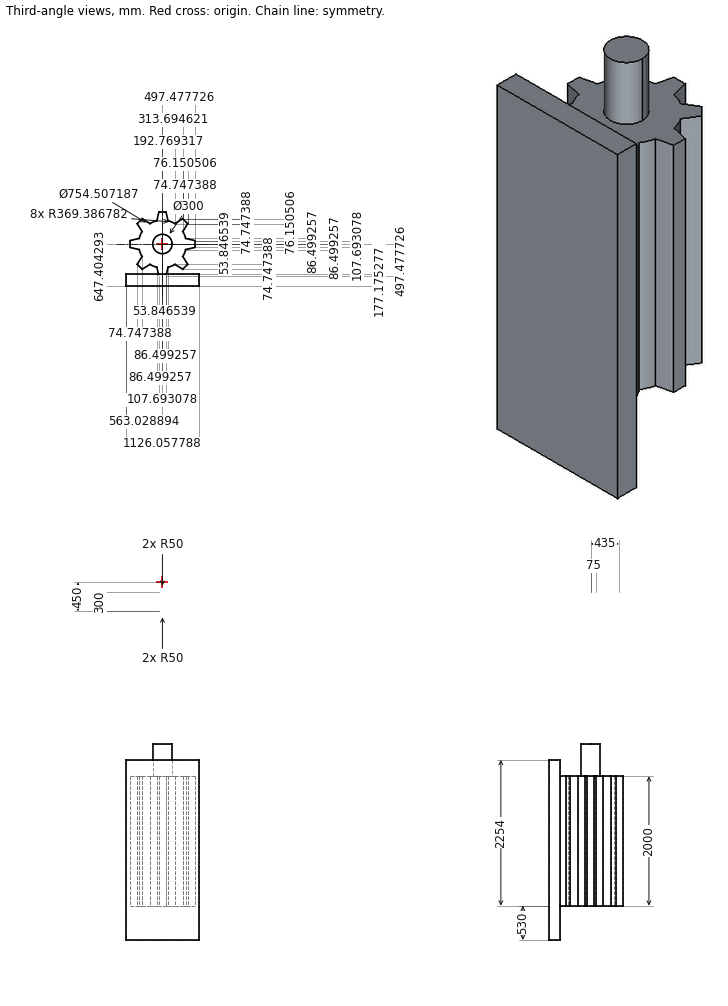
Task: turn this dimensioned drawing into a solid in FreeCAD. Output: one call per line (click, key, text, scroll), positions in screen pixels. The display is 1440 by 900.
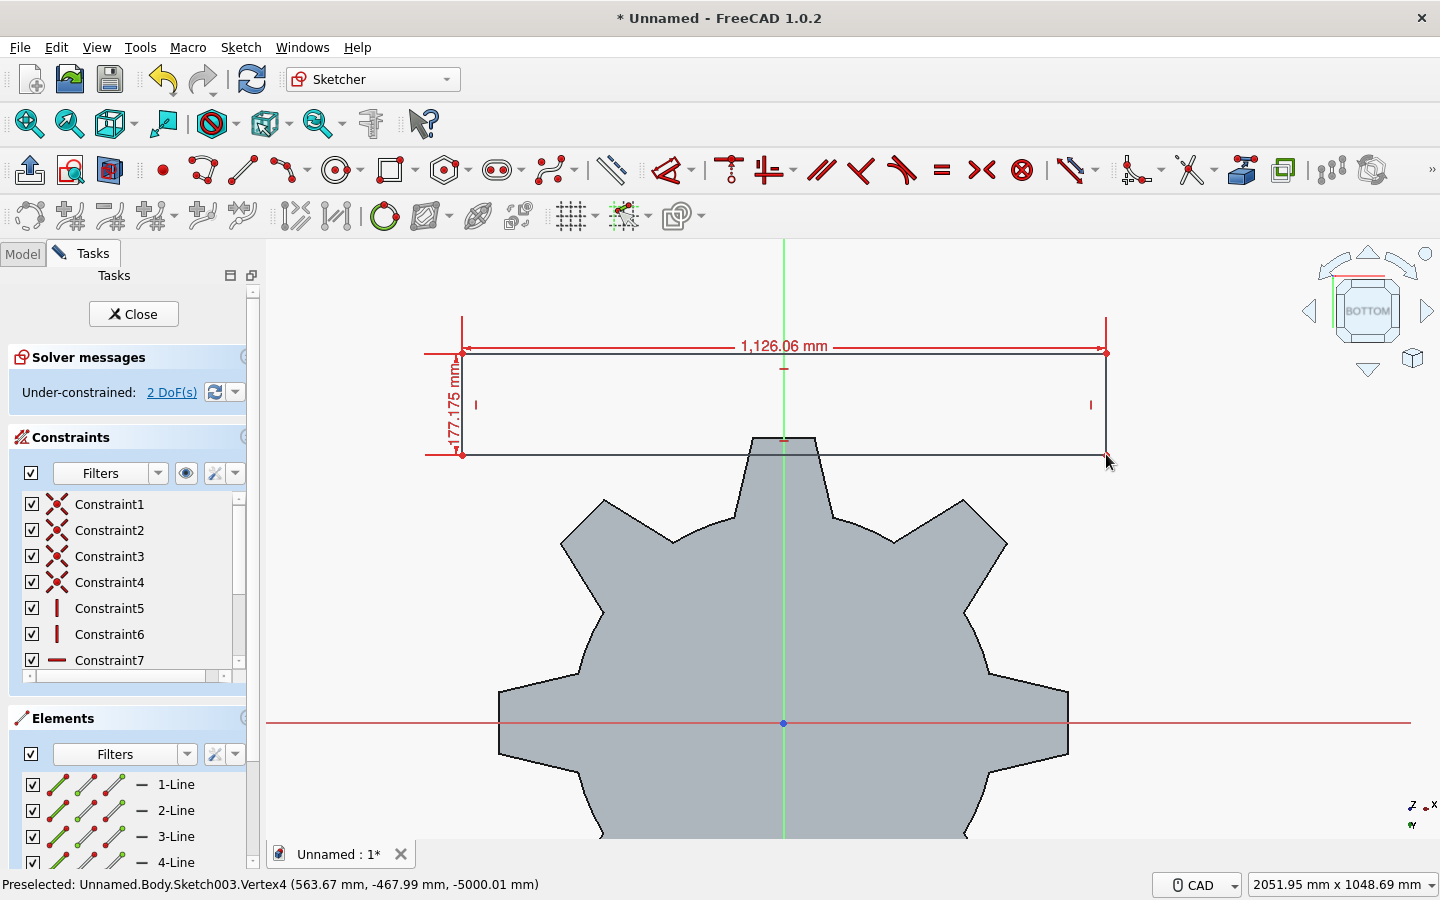
click(666, 170)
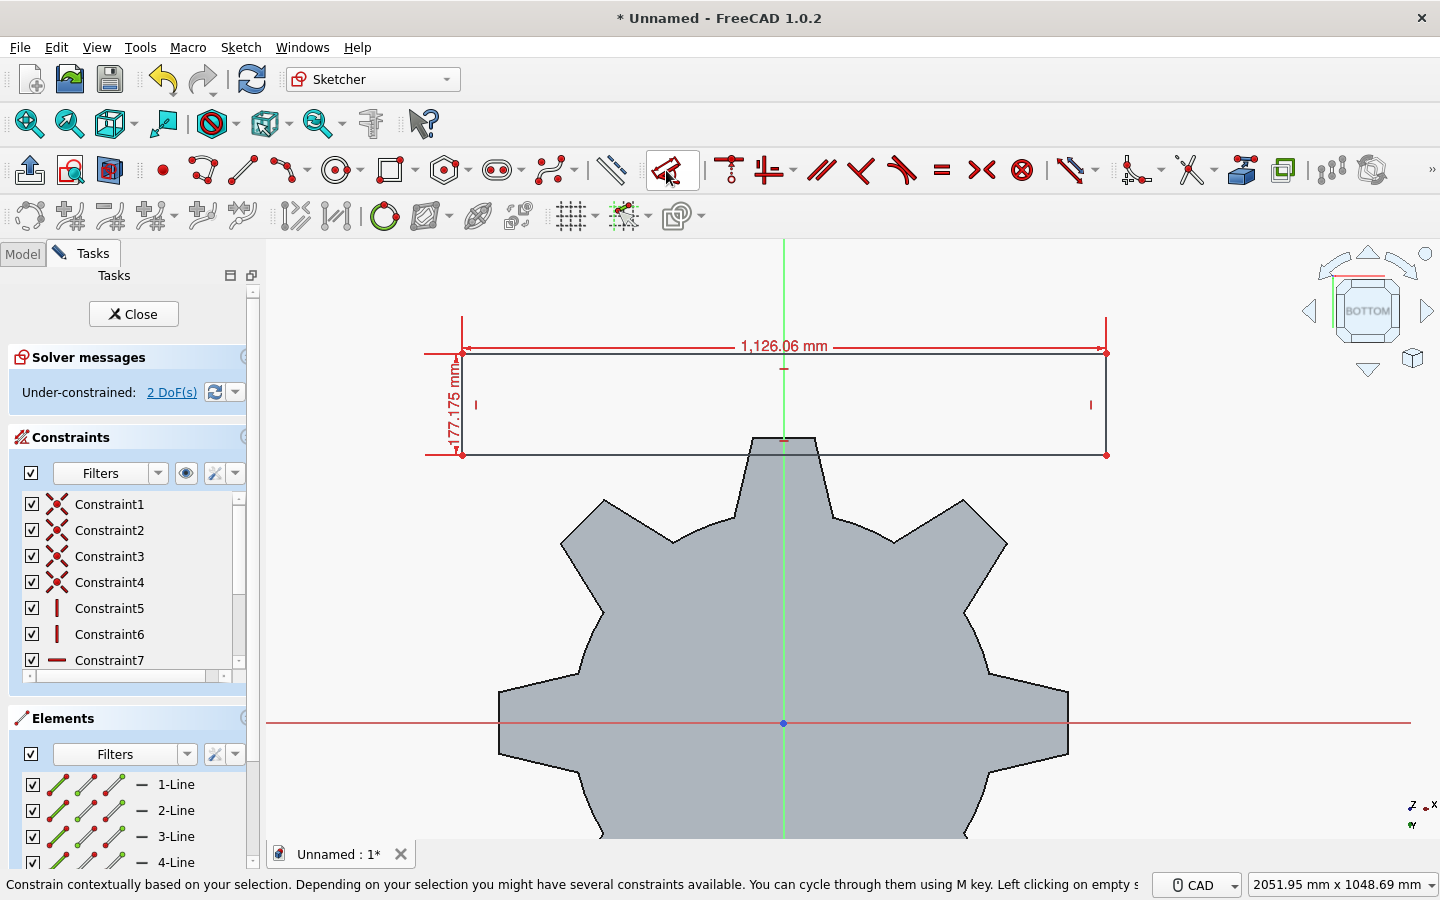
click(462, 354)
click(623, 757)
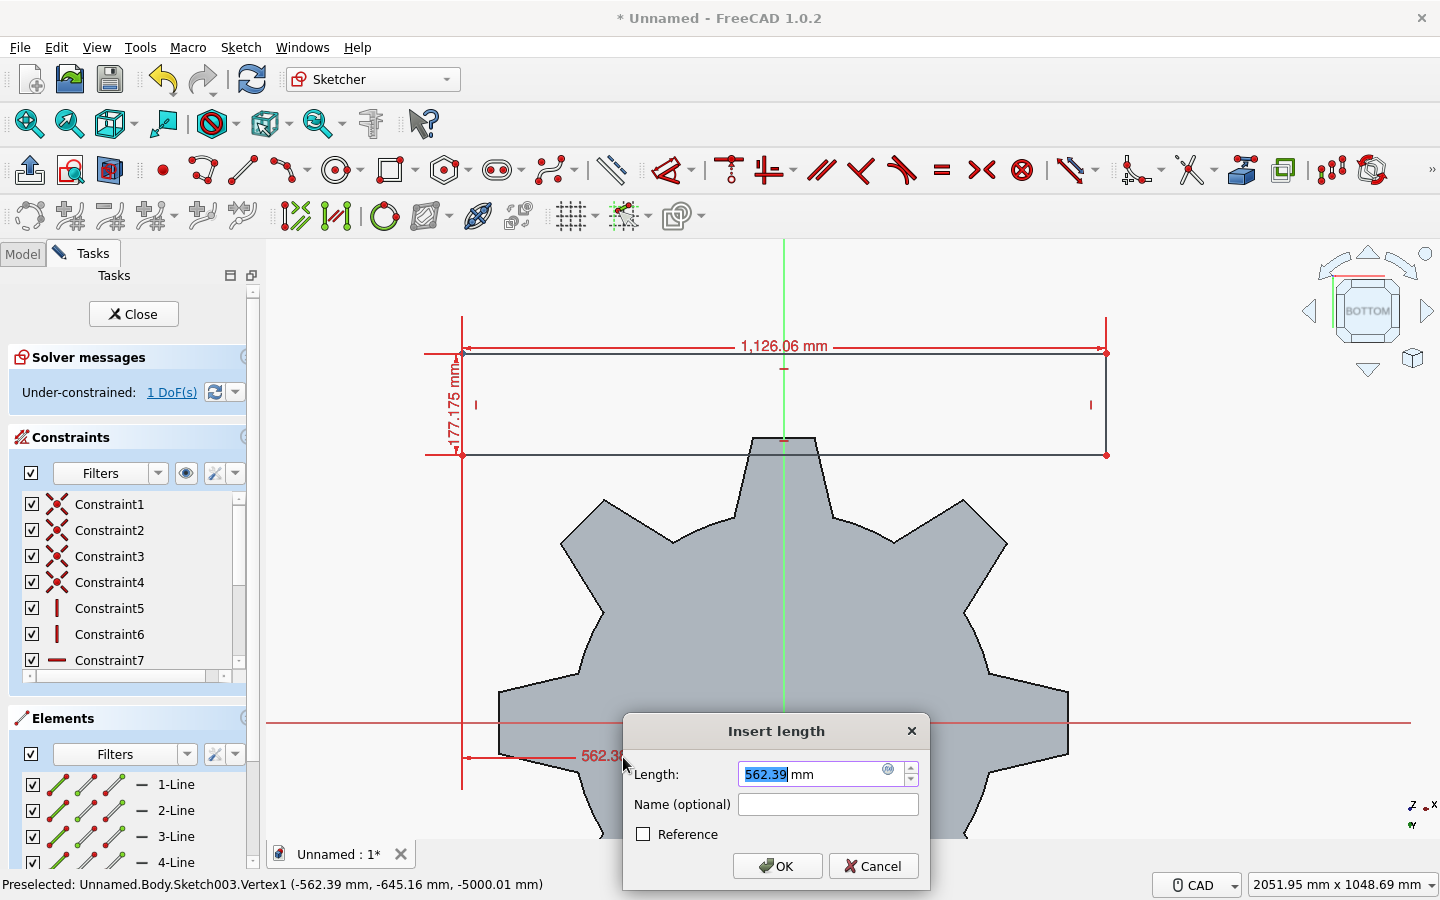
text(563.028894)
key(Return)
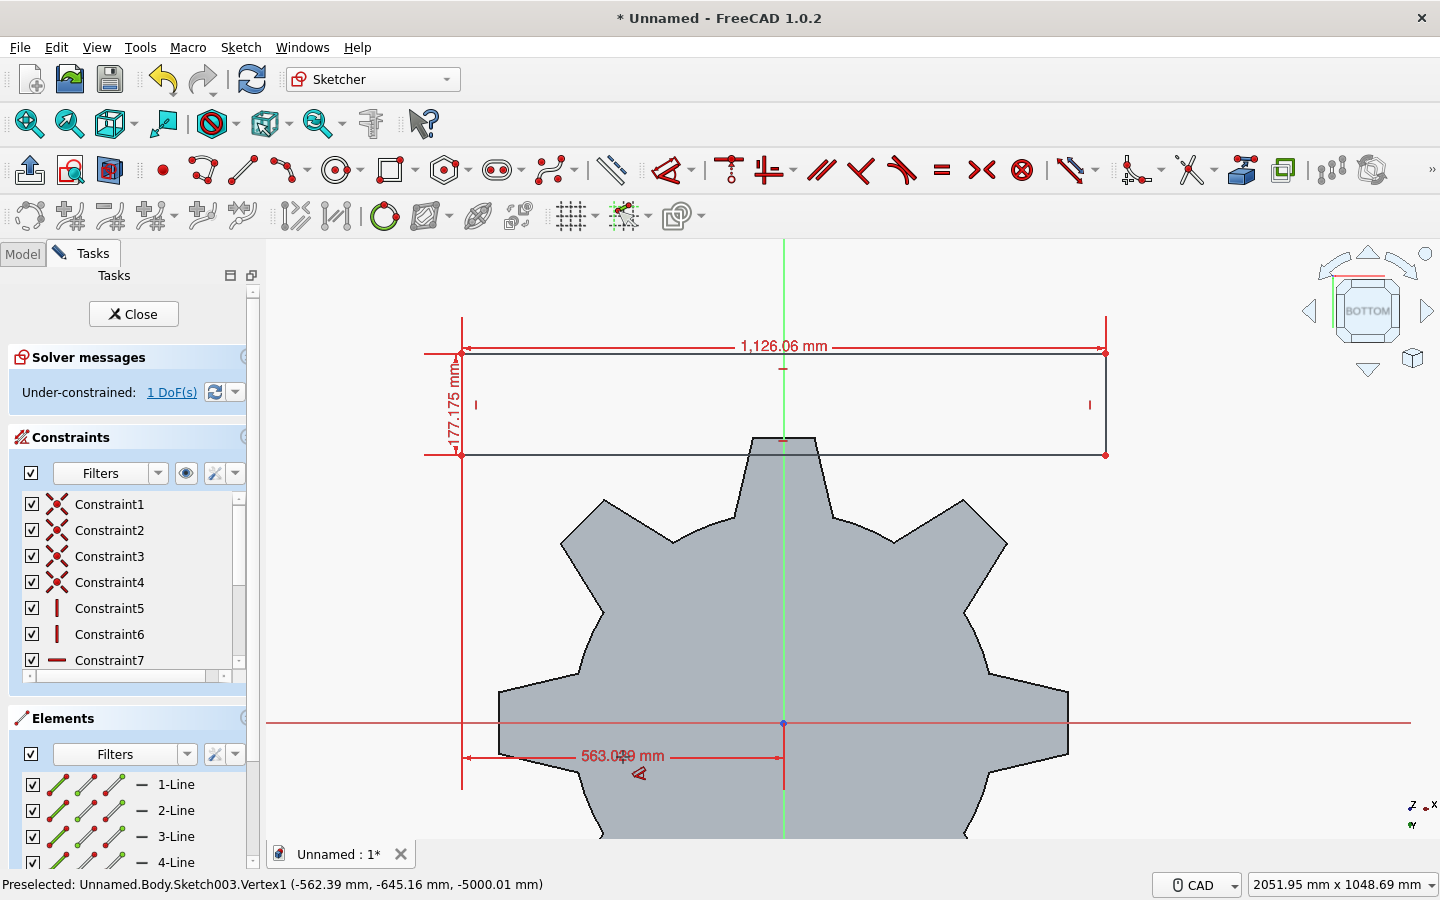
click(462, 354)
click(428, 539)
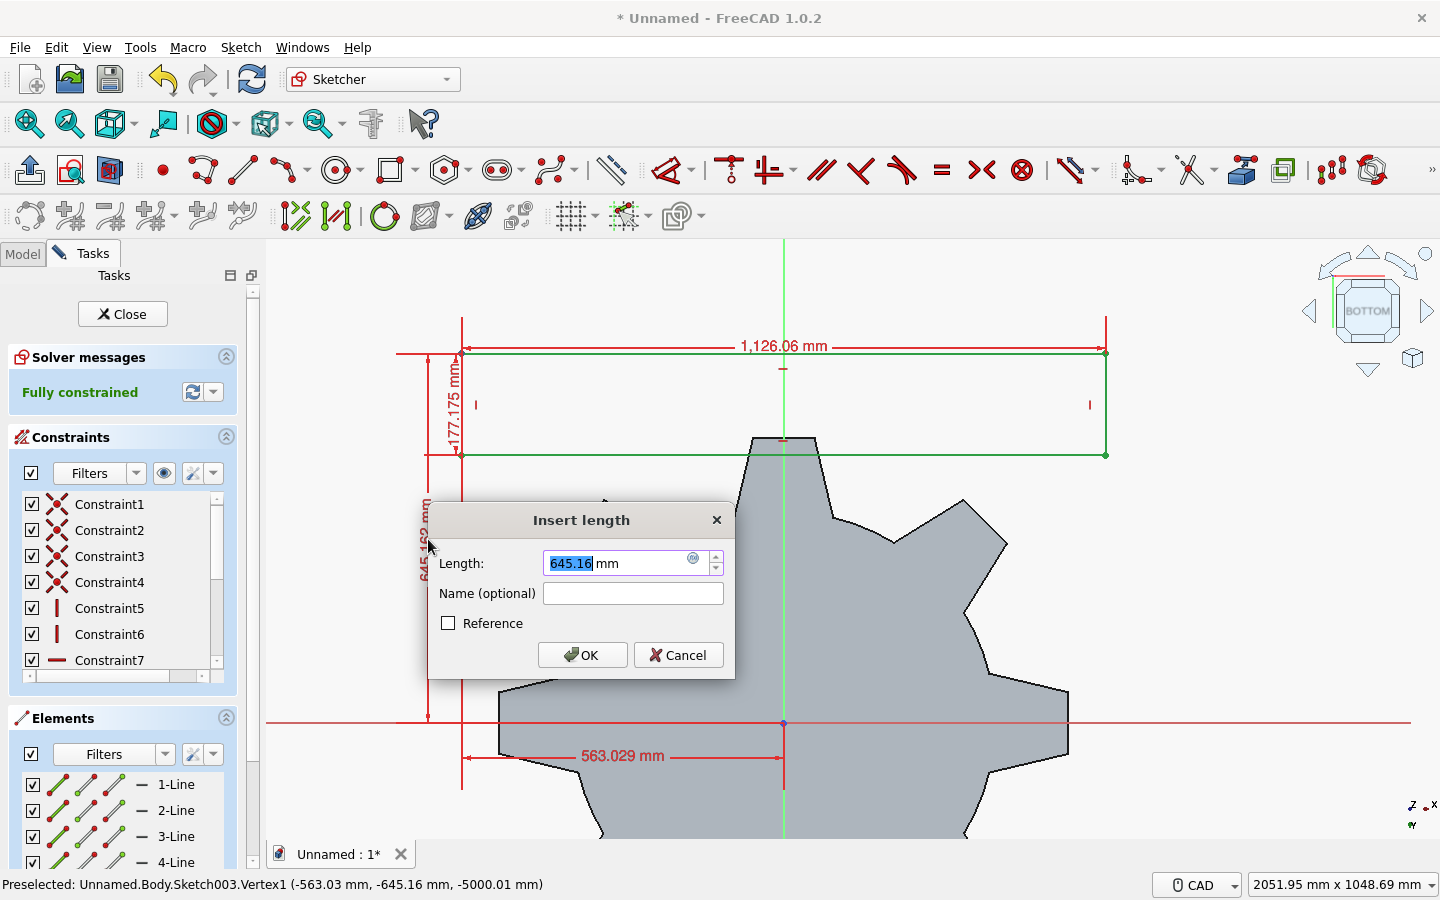
text(647.404293)
key(Return)
key(Escape)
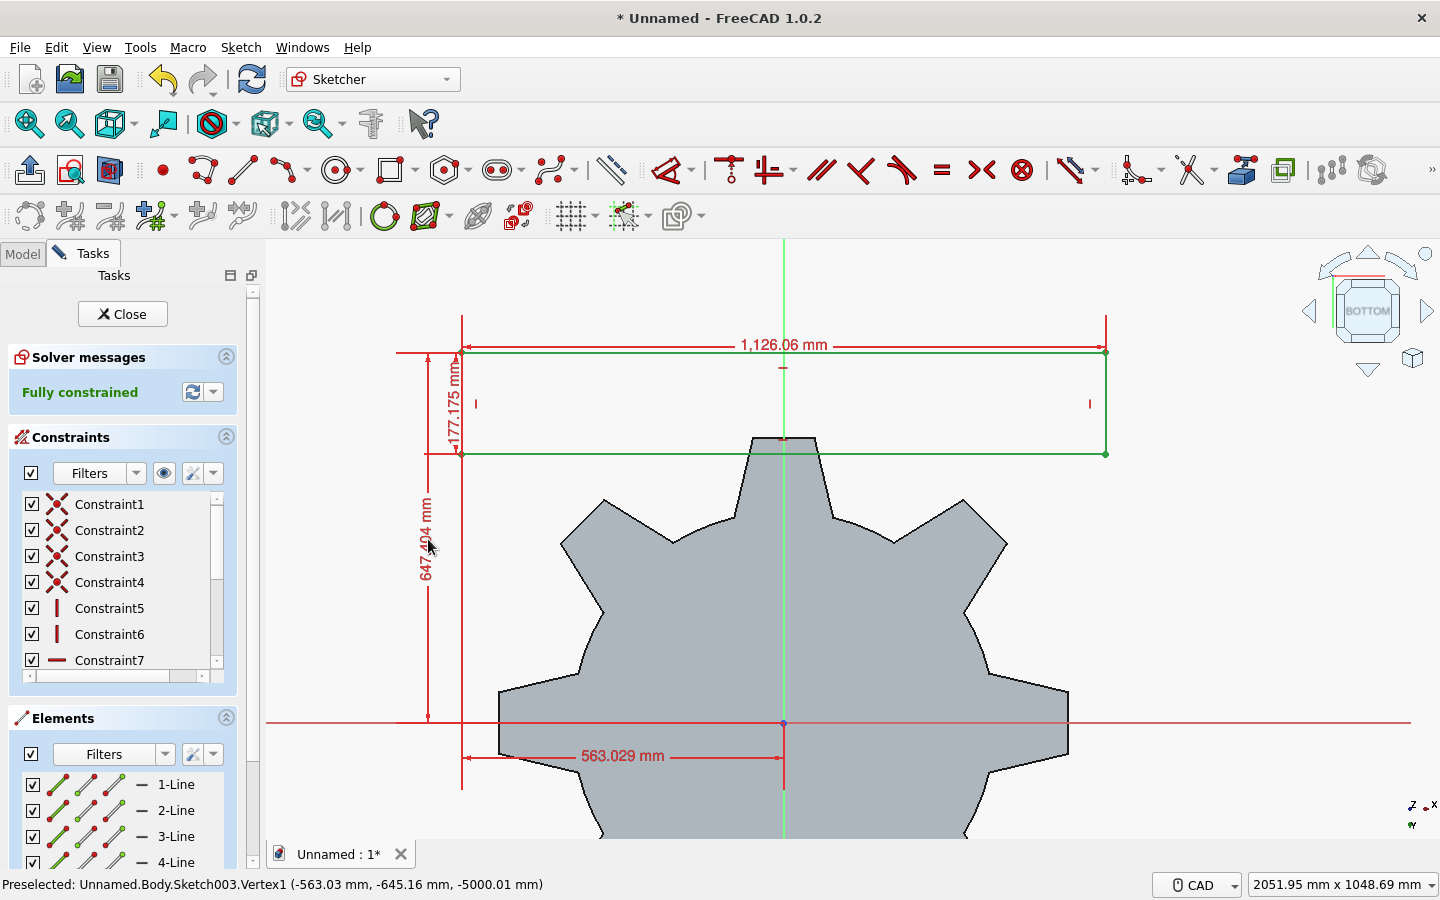
click(123, 314)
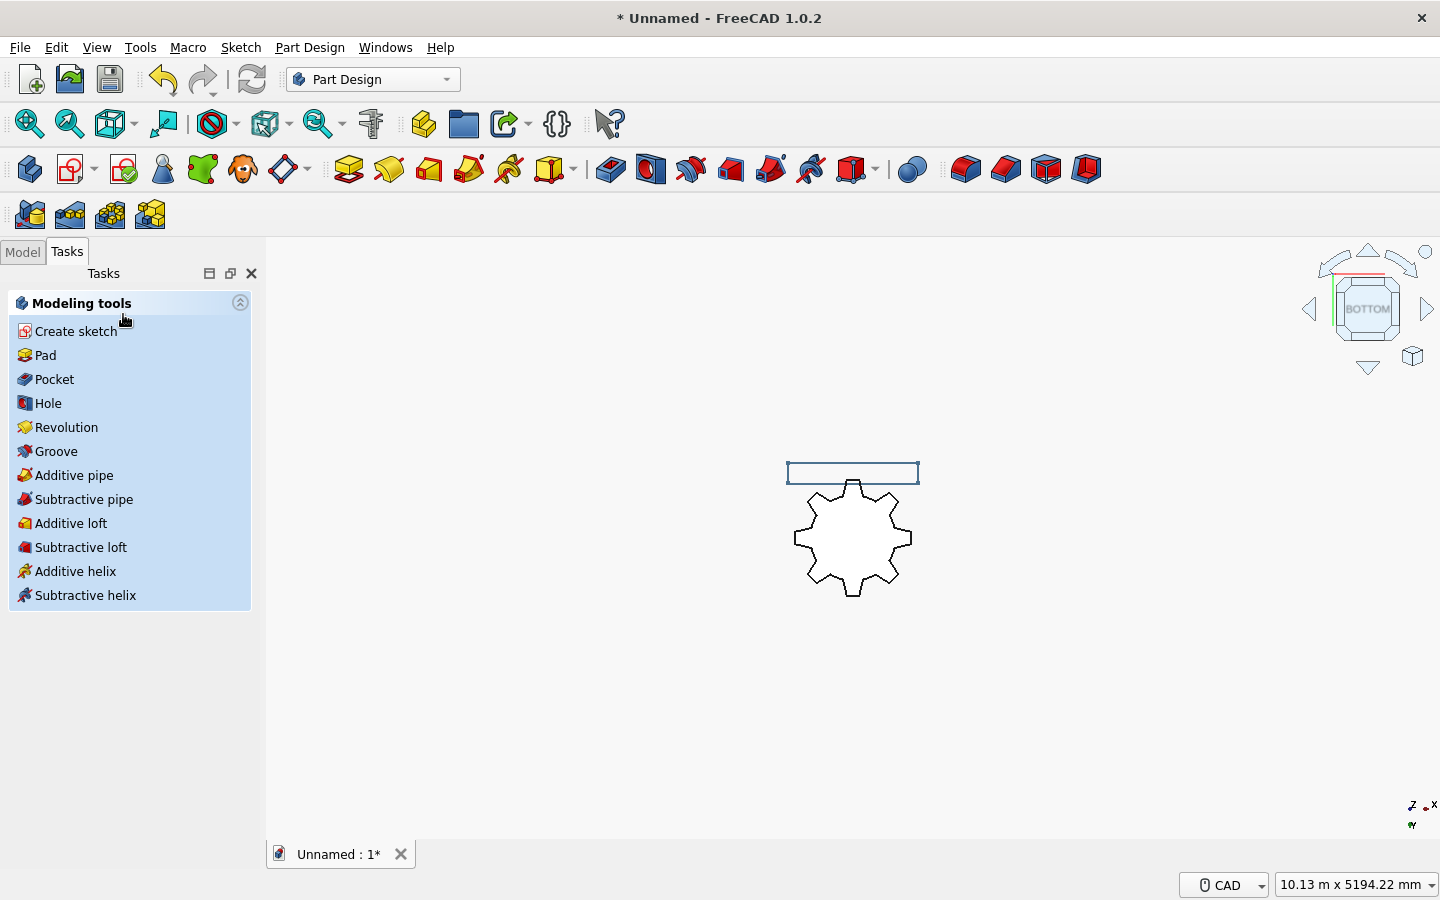
click(350, 170)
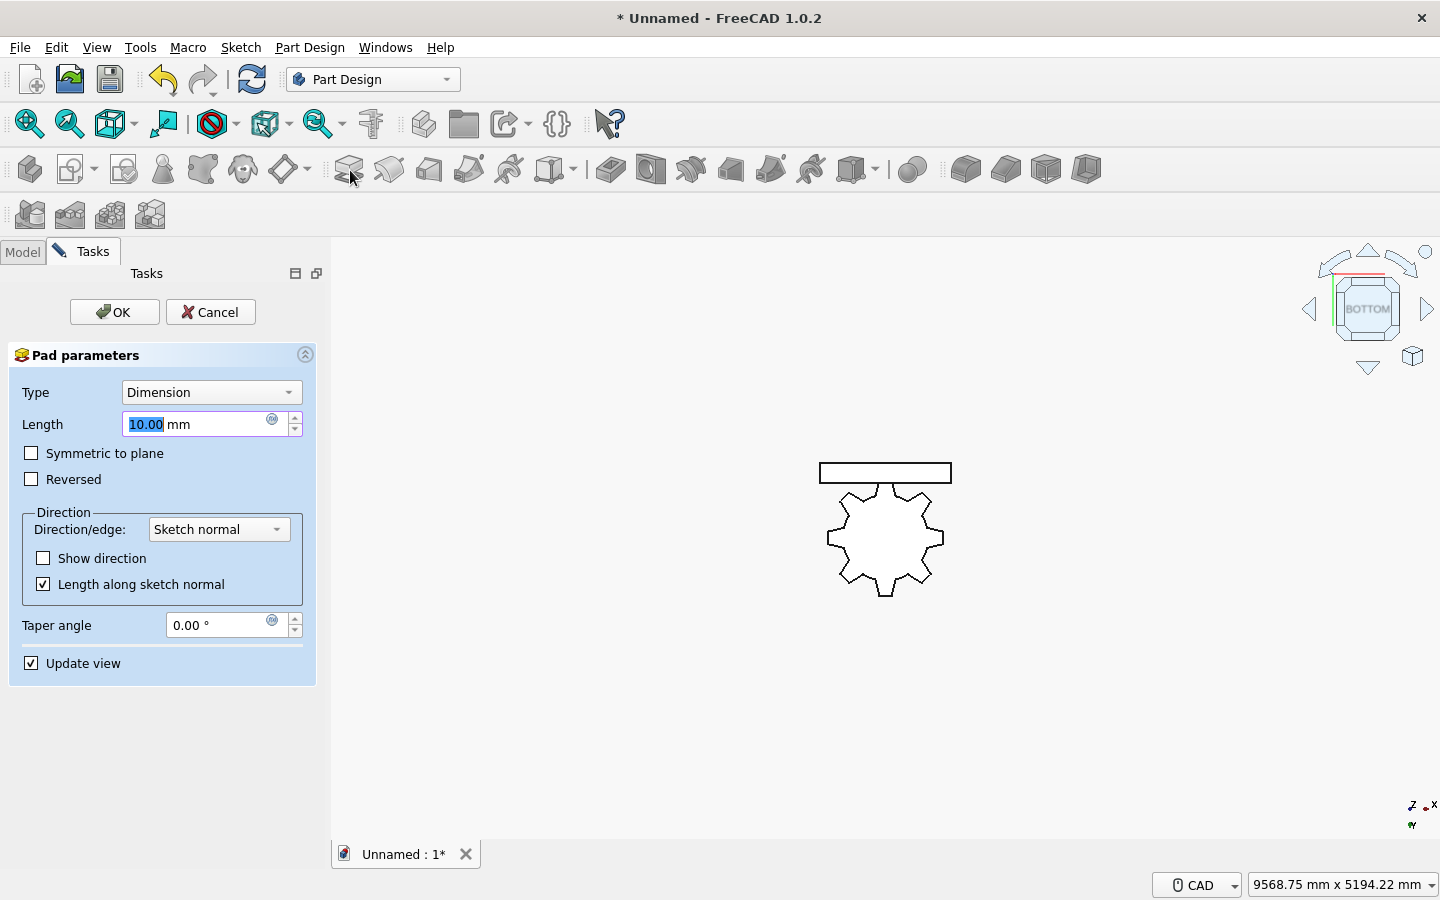
click(212, 392)